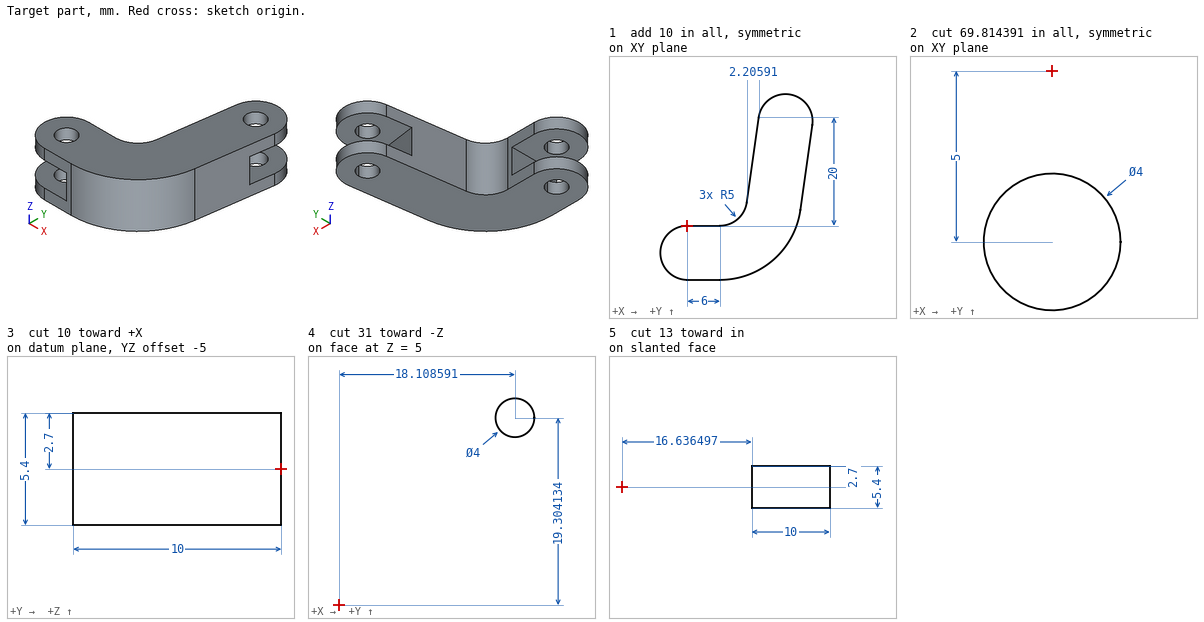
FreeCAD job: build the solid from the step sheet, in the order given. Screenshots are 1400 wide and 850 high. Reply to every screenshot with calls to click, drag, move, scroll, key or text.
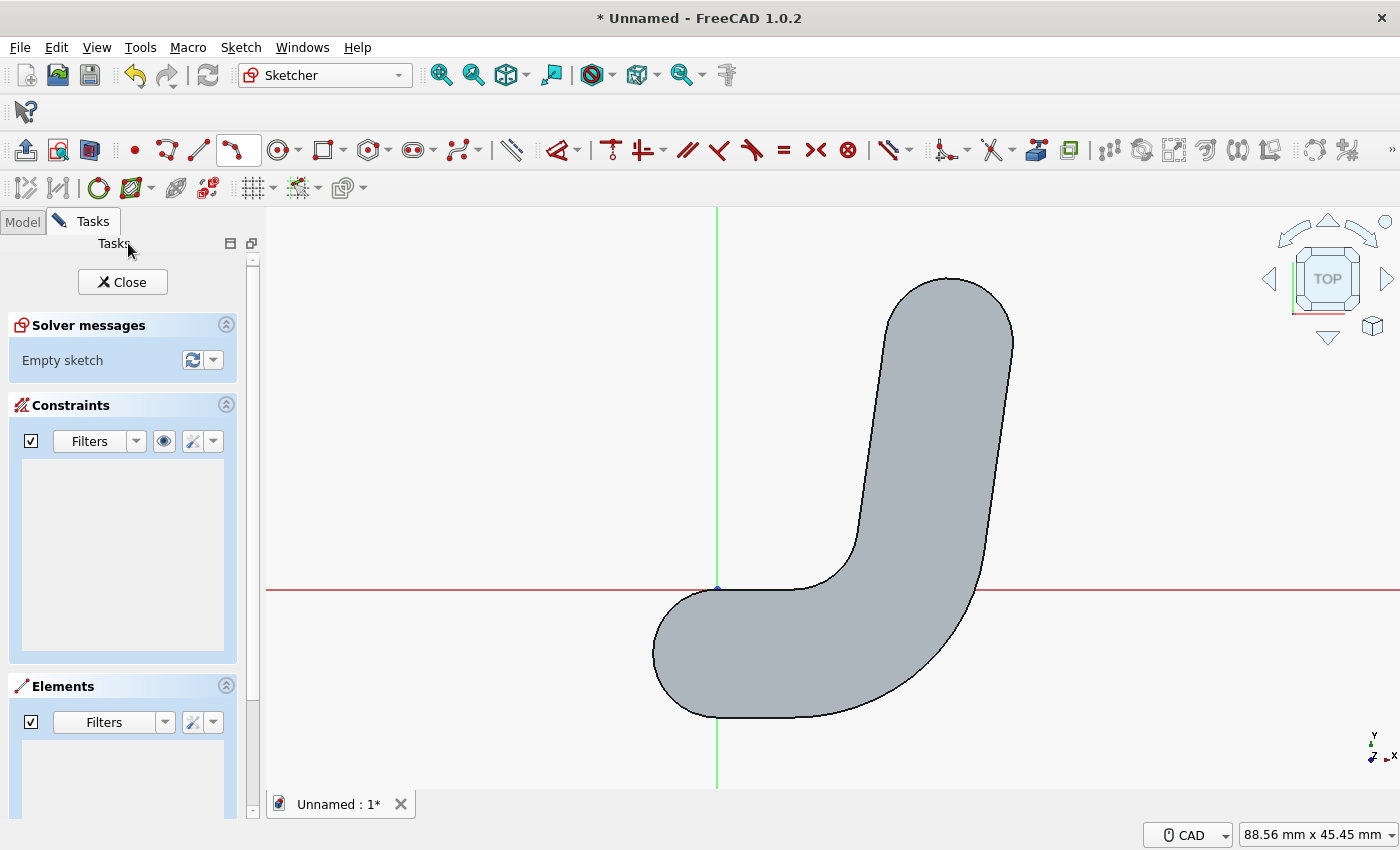
click(90, 150)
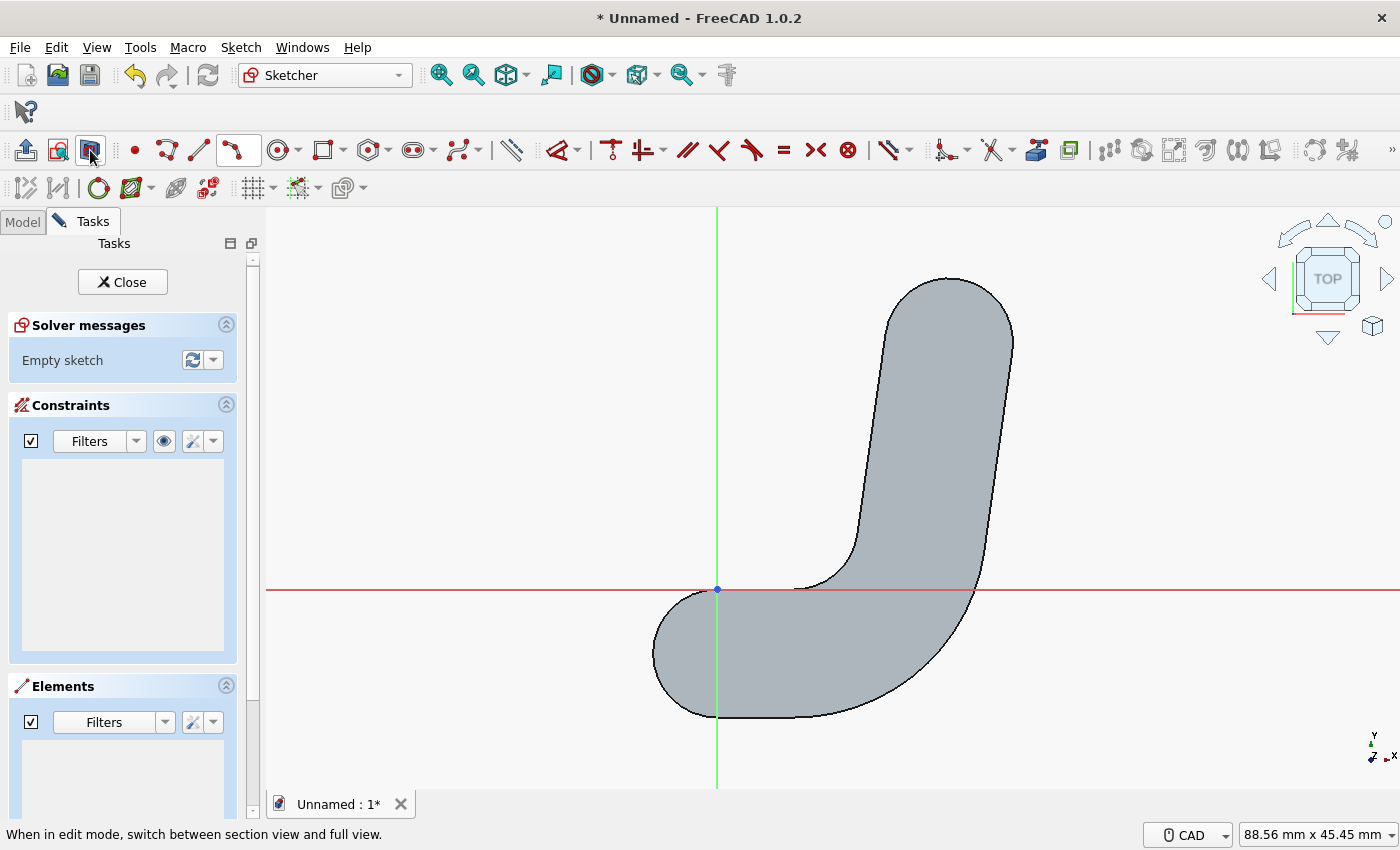
scroll(702, 679, up, 7)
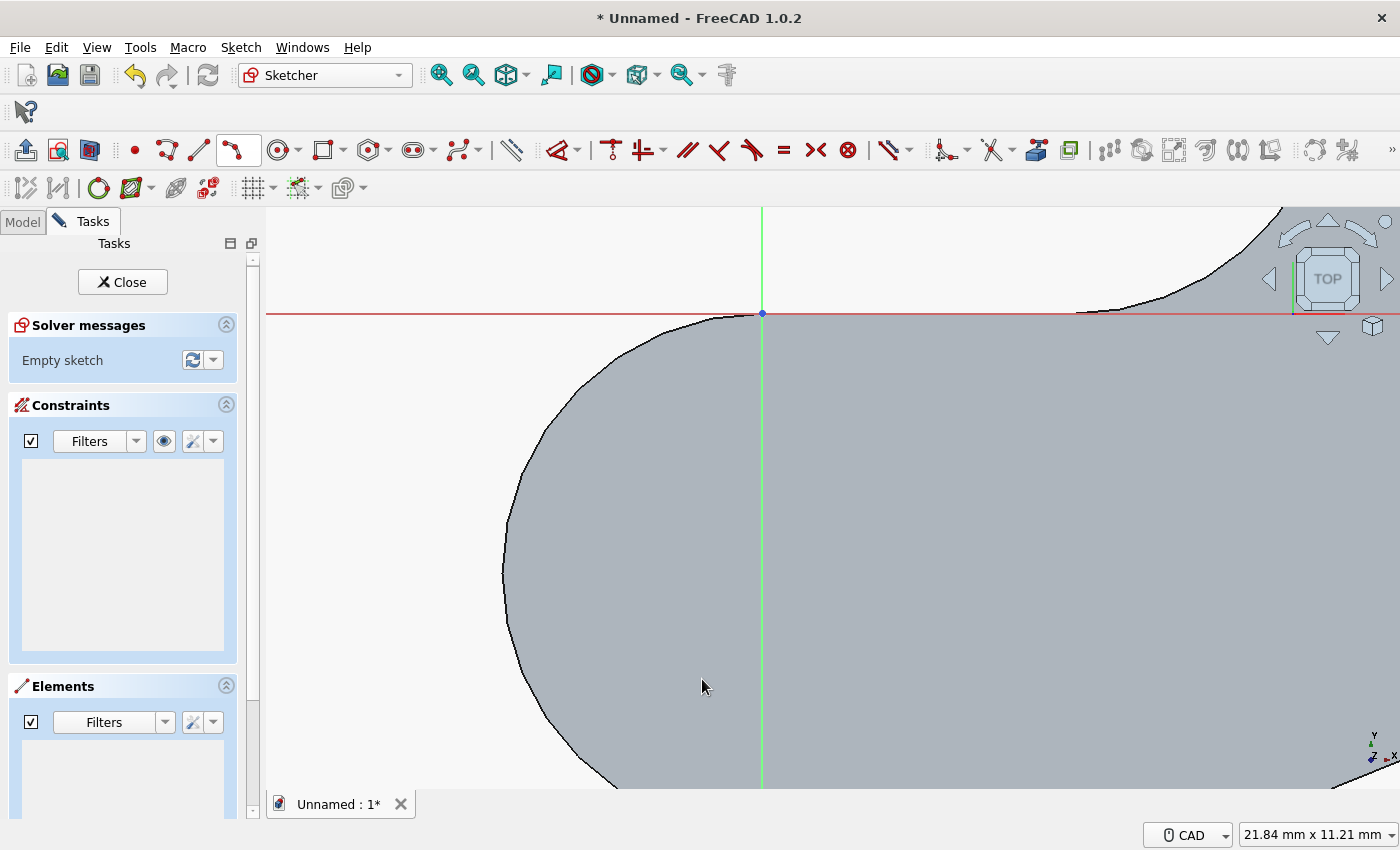
click(278, 150)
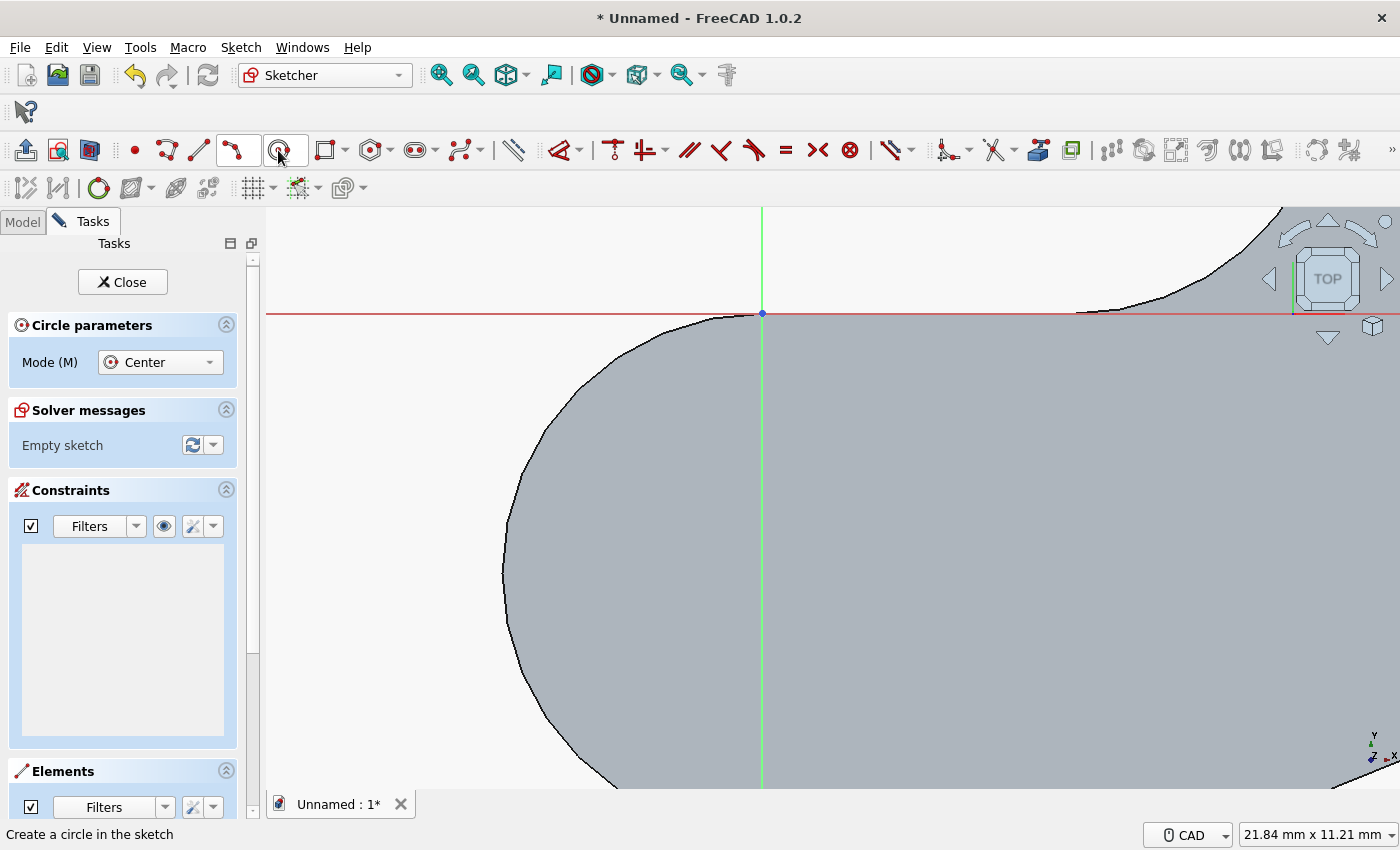
click(762, 573)
click(836, 500)
key(Escape)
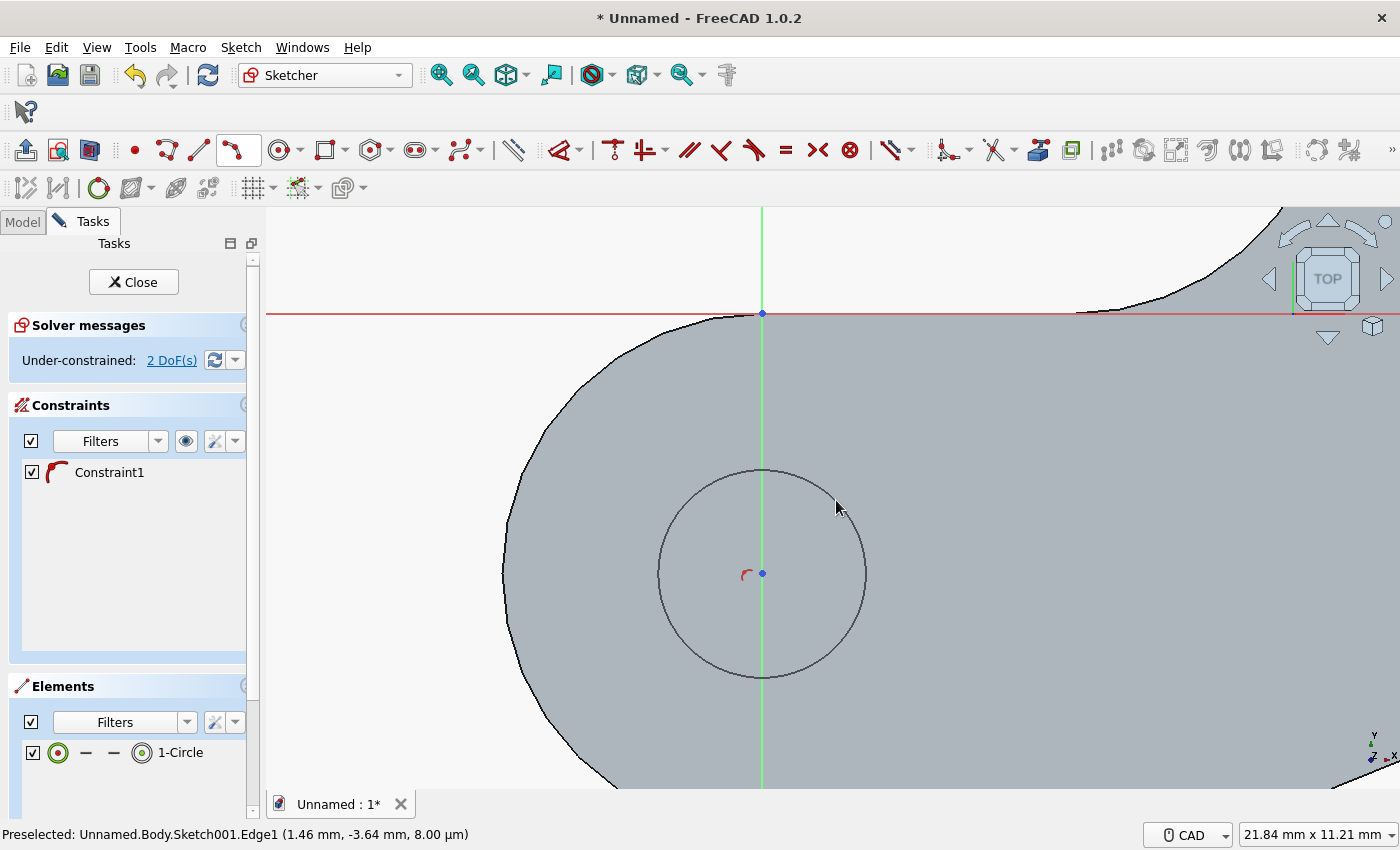
click(560, 150)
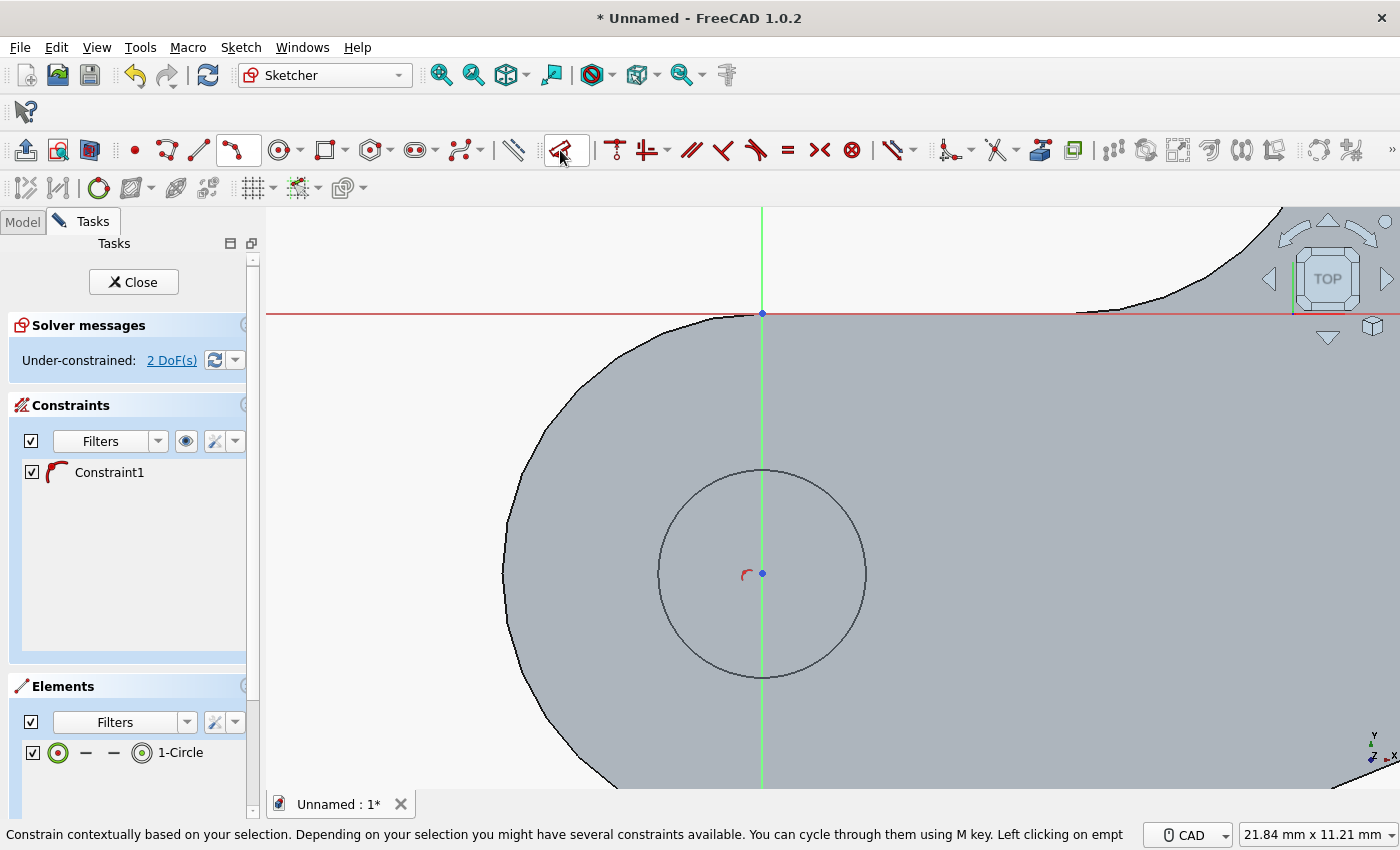
click(835, 500)
click(857, 477)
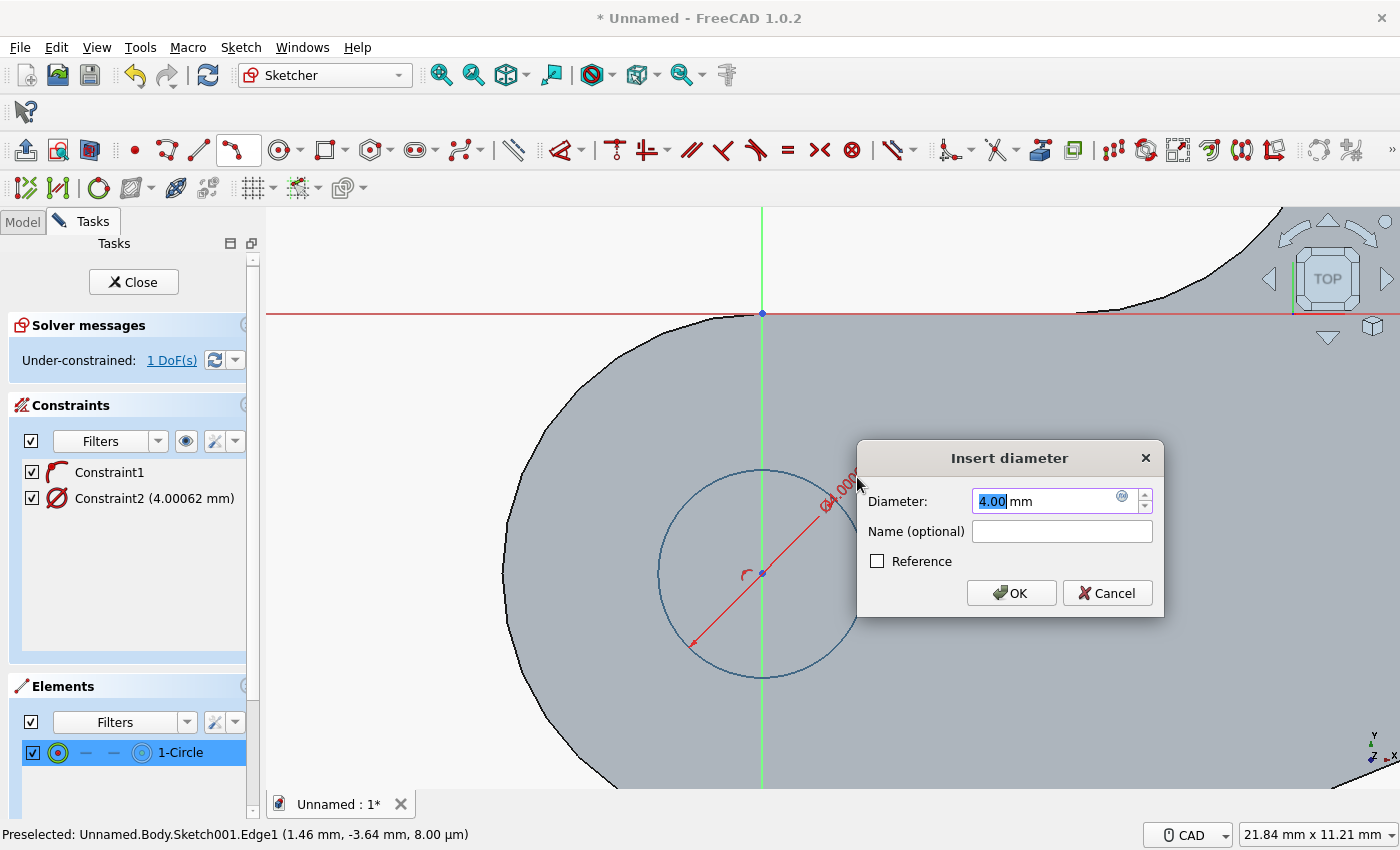
text(4)
key(Return)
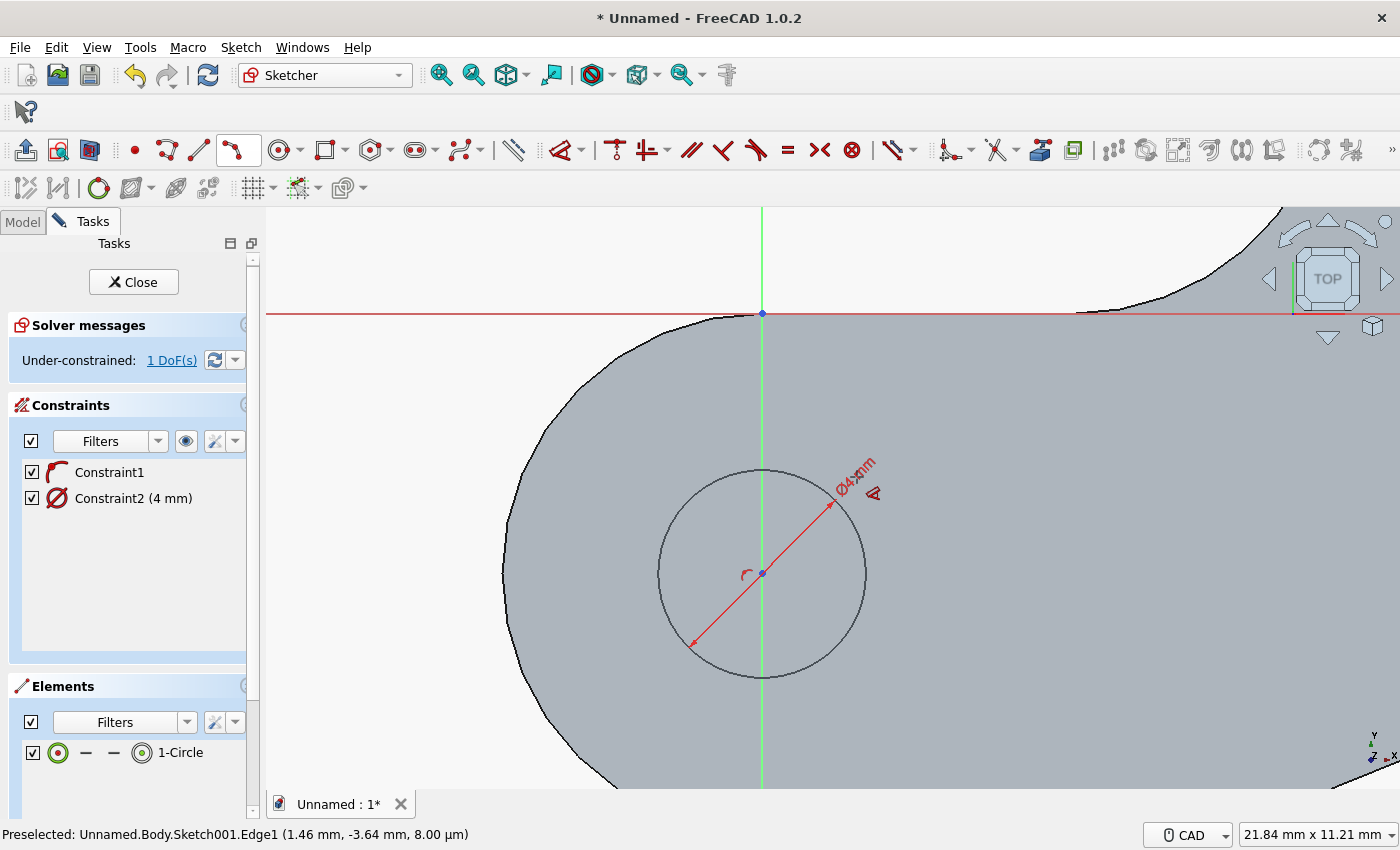
click(762, 574)
click(796, 444)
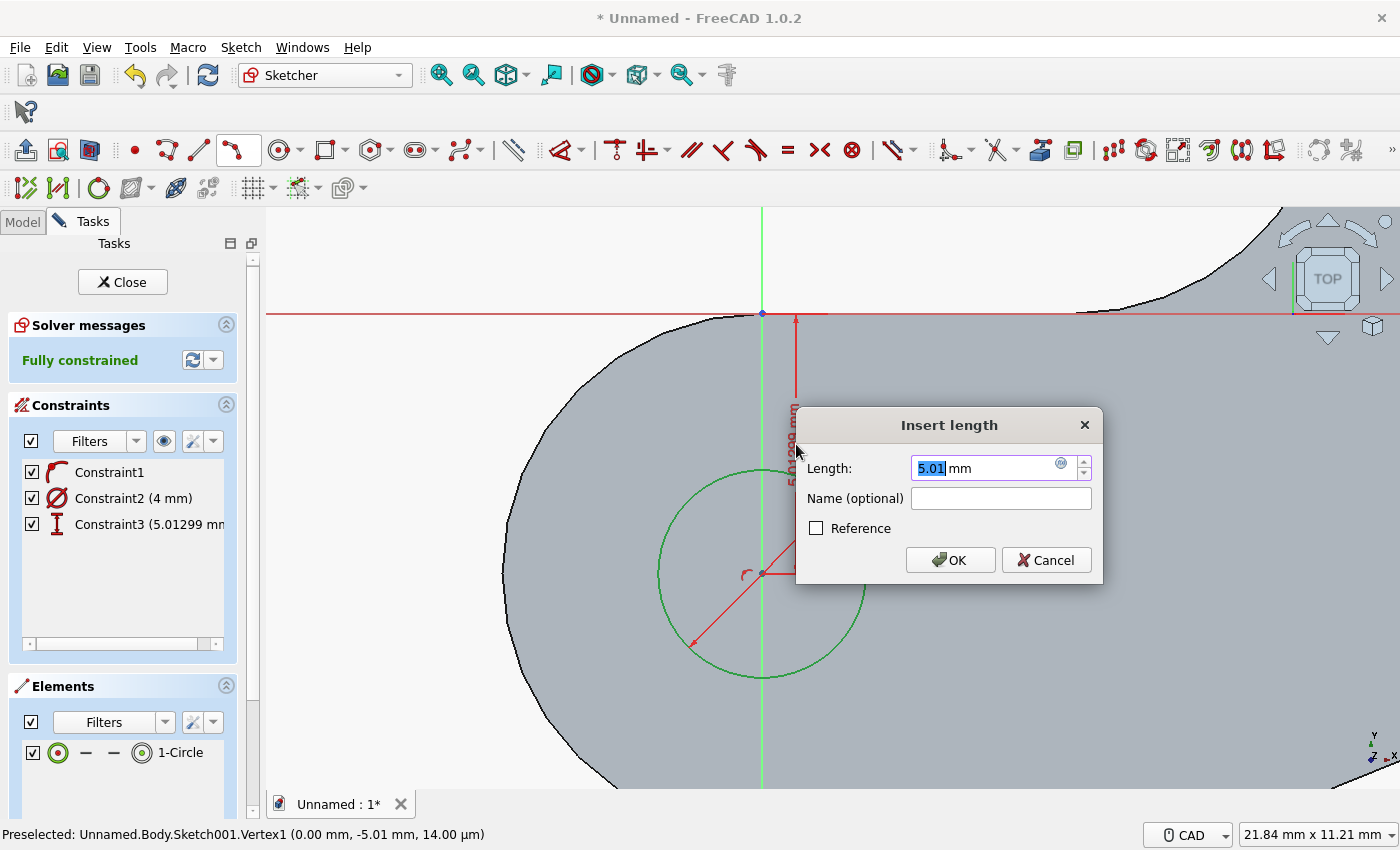
text(5)
key(Return)
key(Escape)